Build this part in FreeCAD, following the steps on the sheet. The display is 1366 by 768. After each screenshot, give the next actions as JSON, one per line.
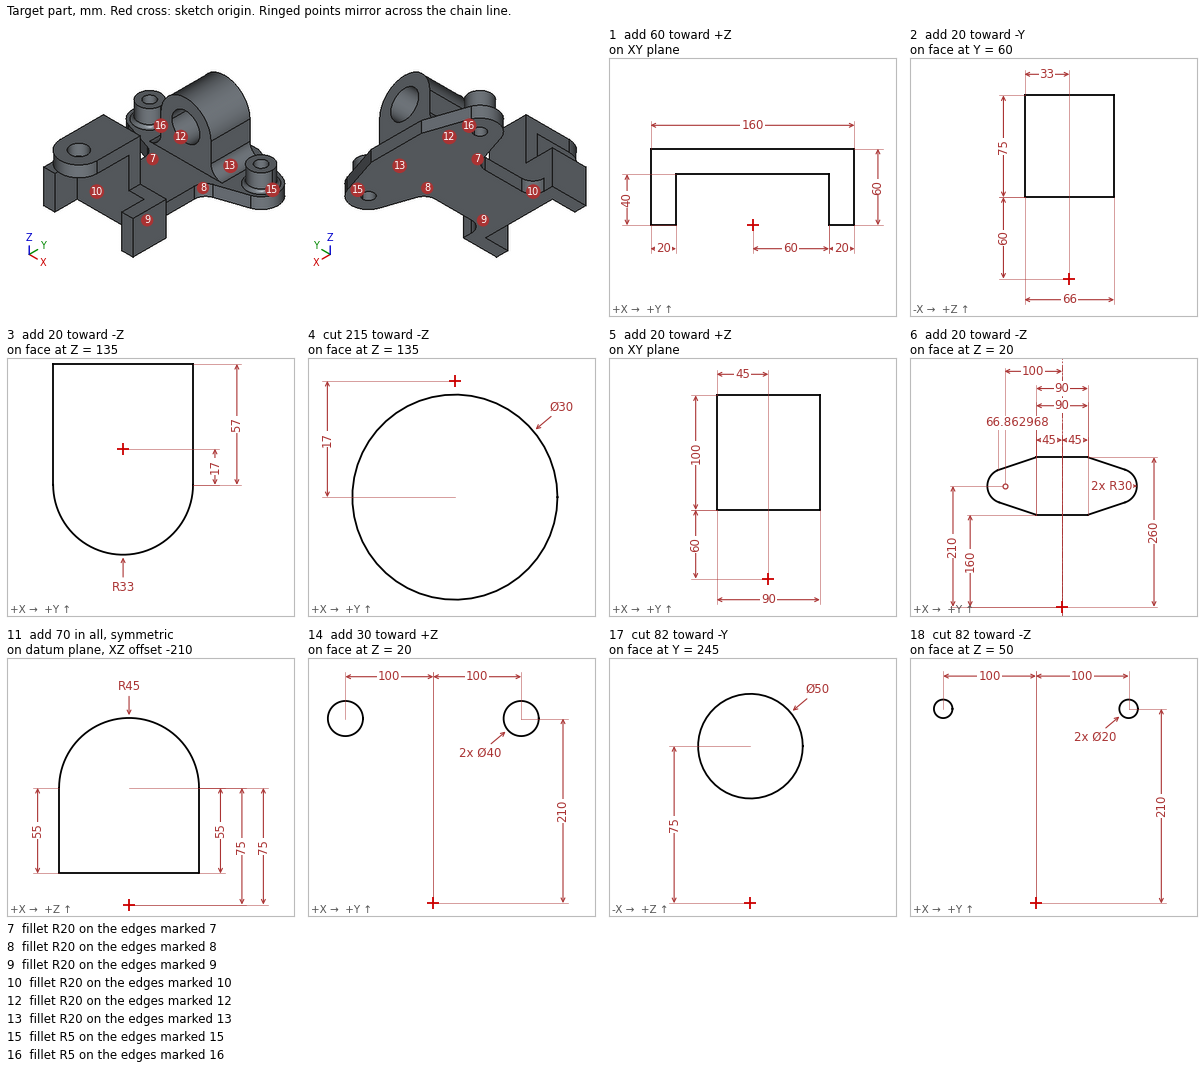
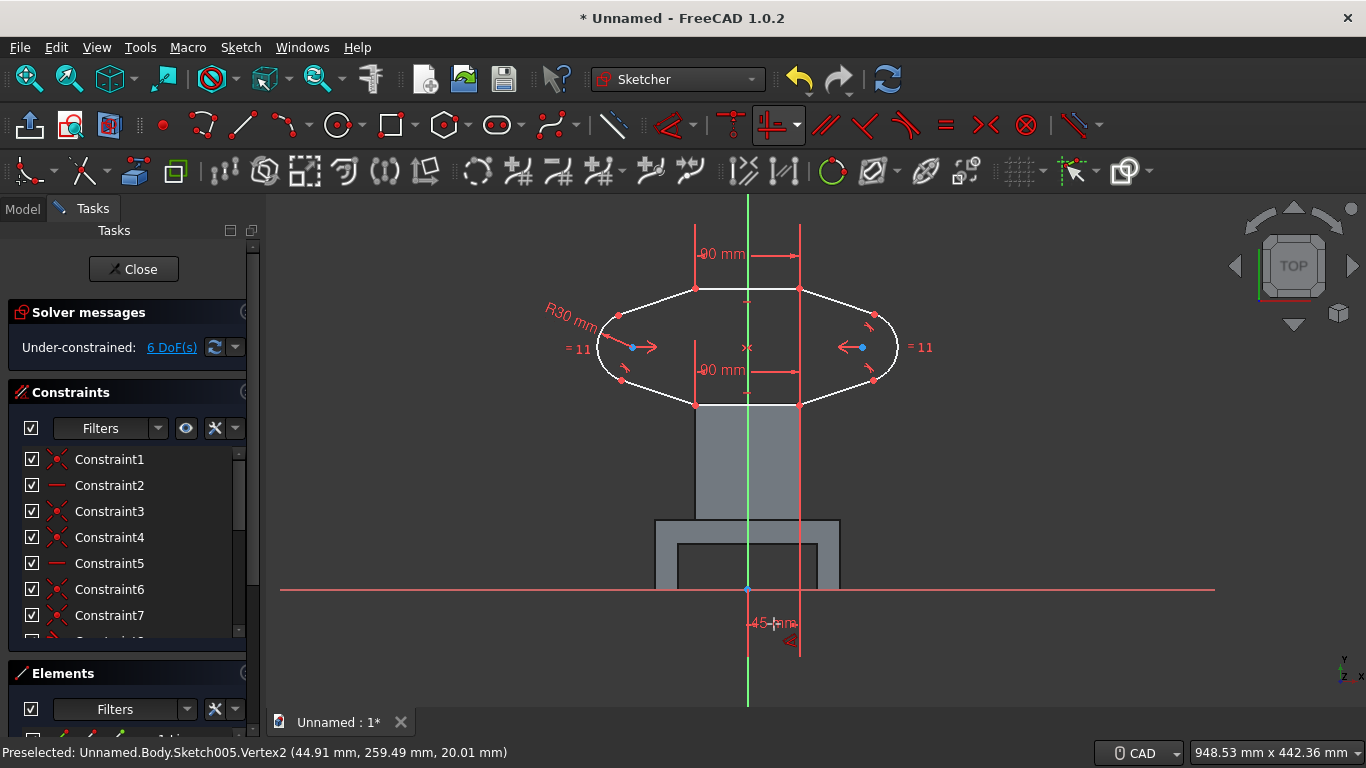
{"action": "left_click", "coordinate": [695, 405]}
{"action": "left_click", "coordinate": [703, 624]}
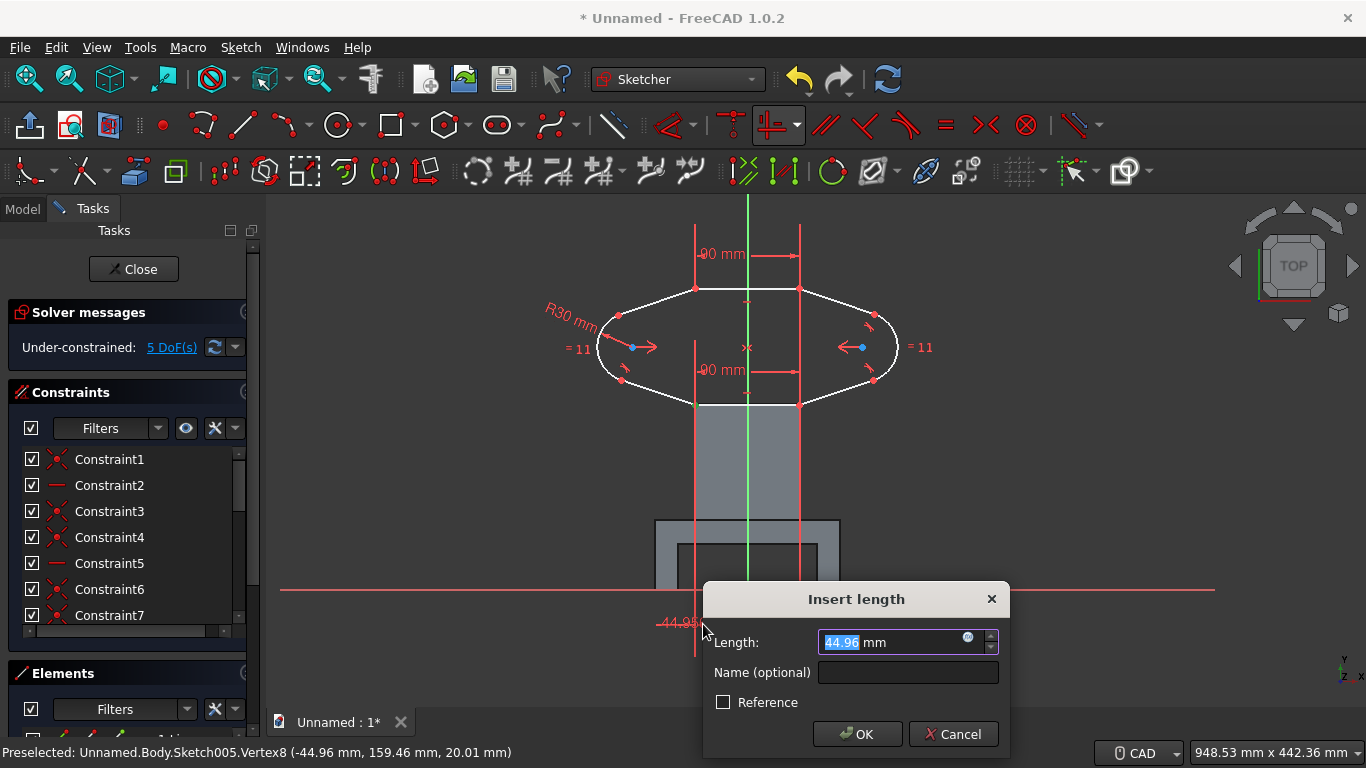
{"action": "type", "text": "45"}
{"action": "key", "text": "Return"}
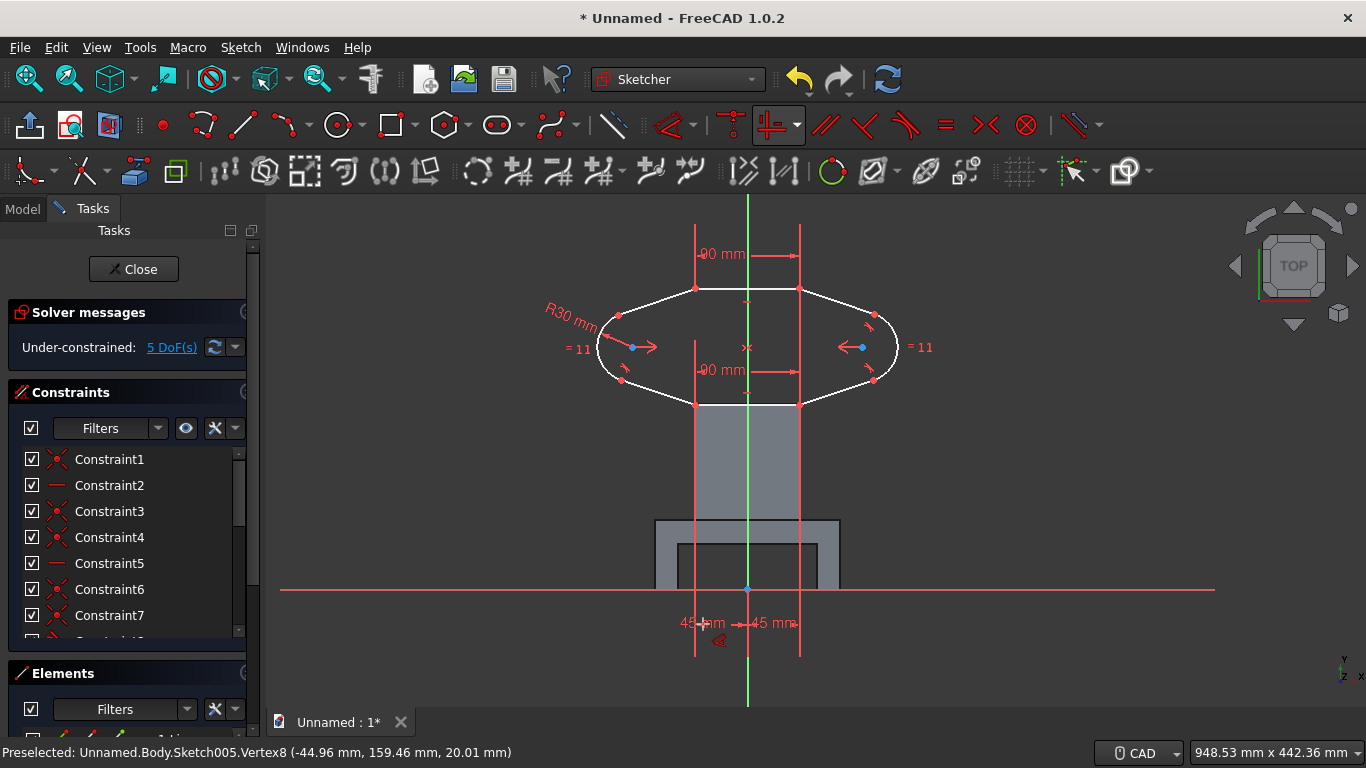
{"action": "left_click", "coordinate": [800, 289]}
{"action": "left_click", "coordinate": [834, 439]}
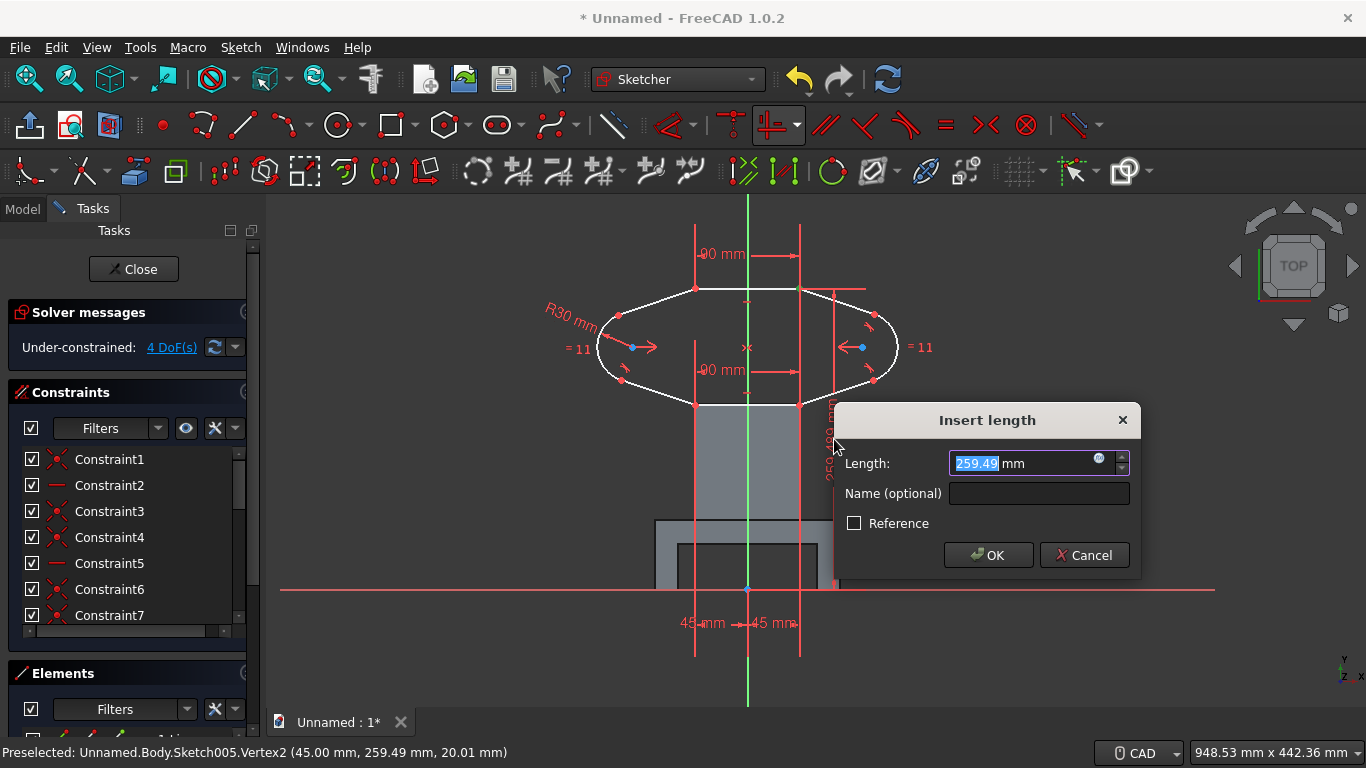
{"action": "type", "text": "260"}
{"action": "key", "text": "Return"}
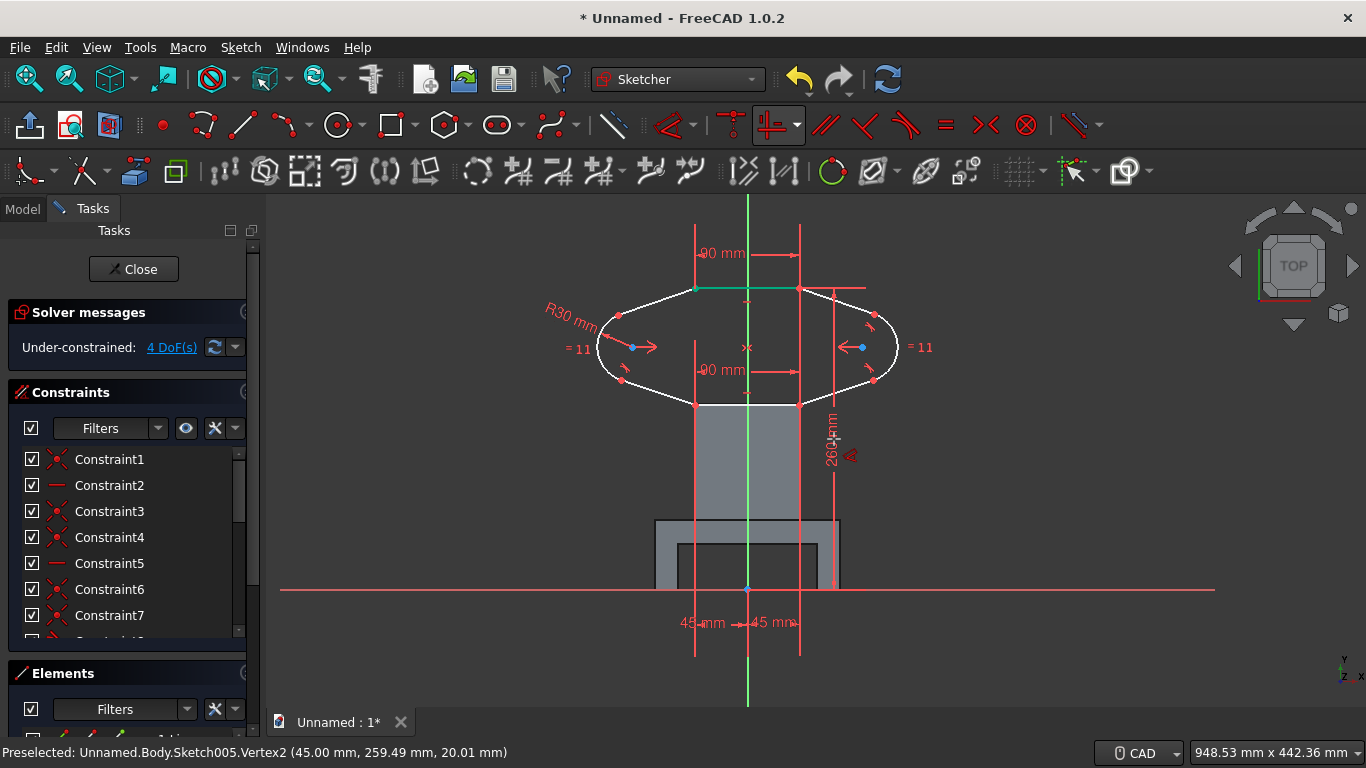
{"action": "left_click", "coordinate": [695, 405]}
{"action": "left_click", "coordinate": [661, 497]}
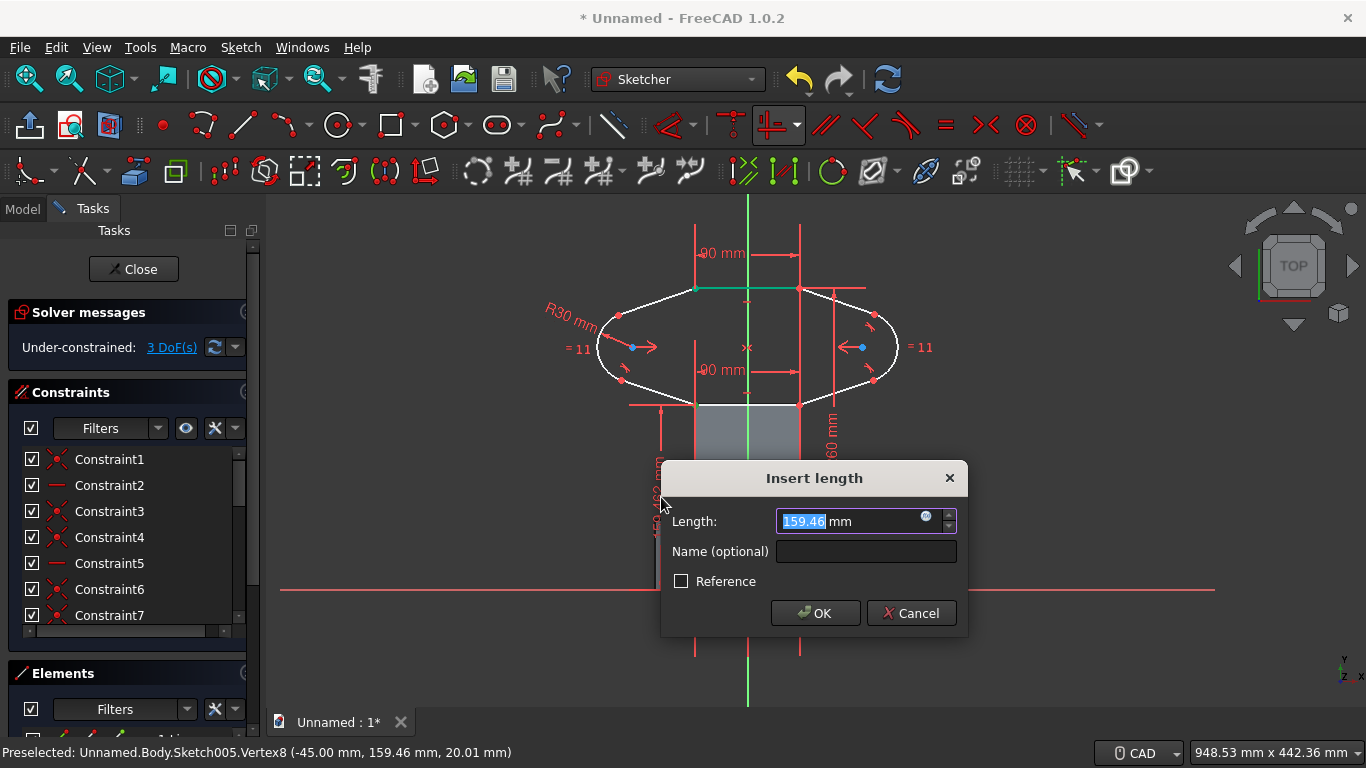
{"action": "type", "text": "160"}
{"action": "key", "text": "Return"}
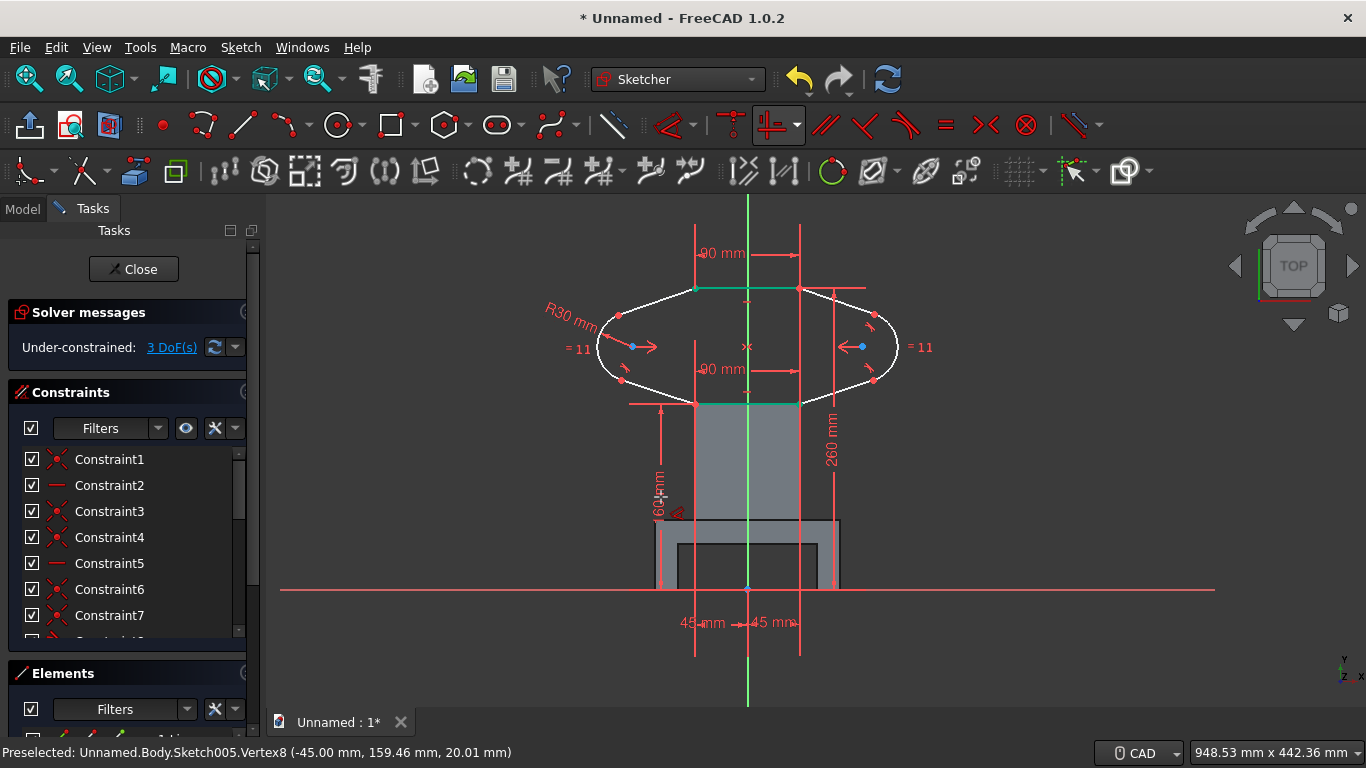
{"action": "left_click", "coordinate": [632, 347]}
{"action": "left_click", "coordinate": [690, 313]}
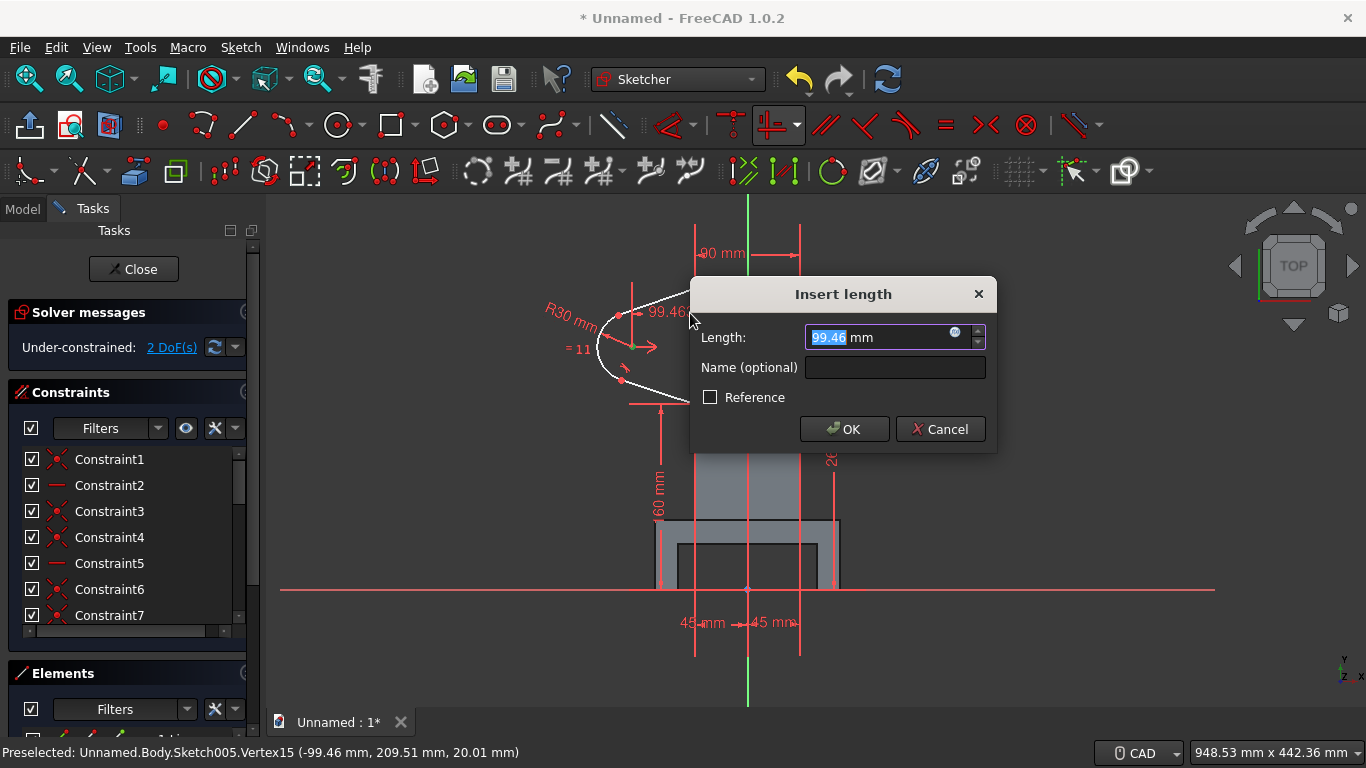
{"action": "type", "text": "100"}
{"action": "key", "text": "Return"}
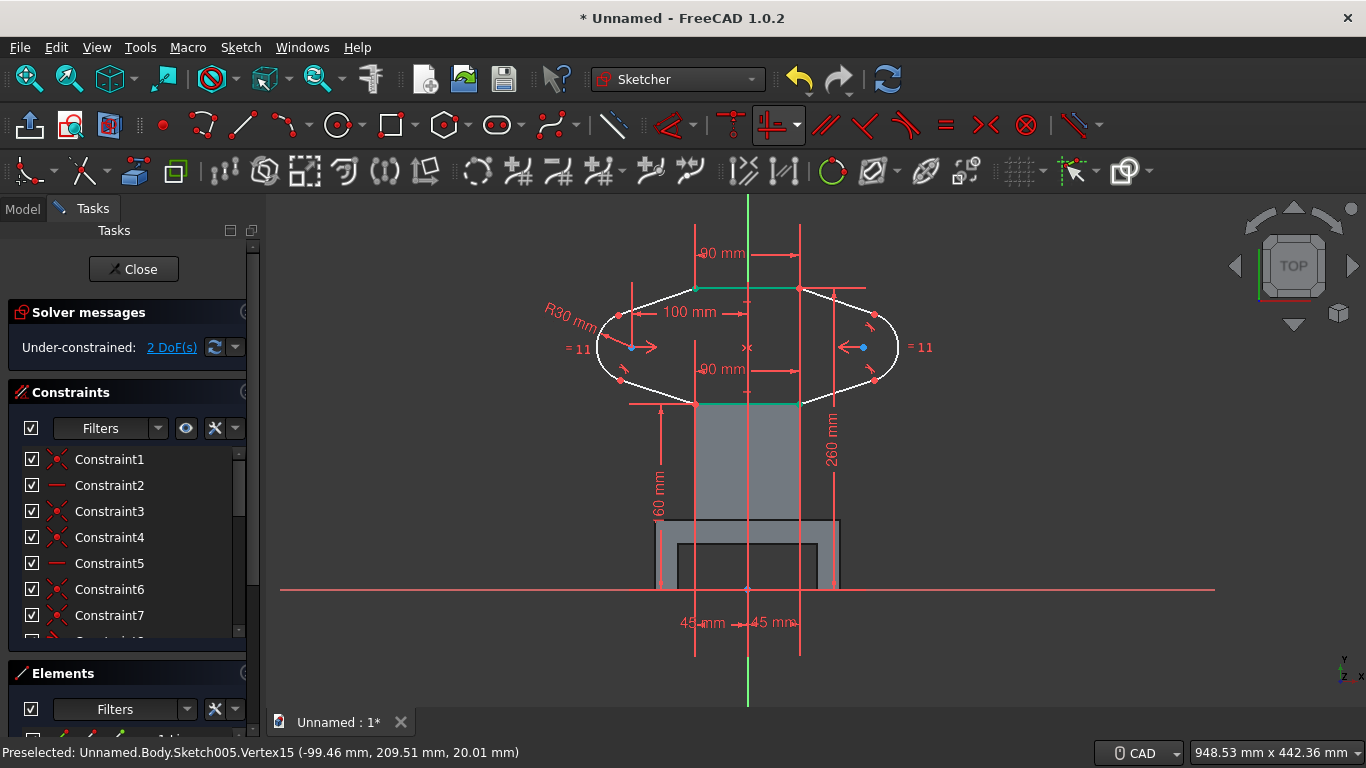
{"action": "left_click", "coordinate": [632, 347]}
{"action": "left_click", "coordinate": [598, 469]}